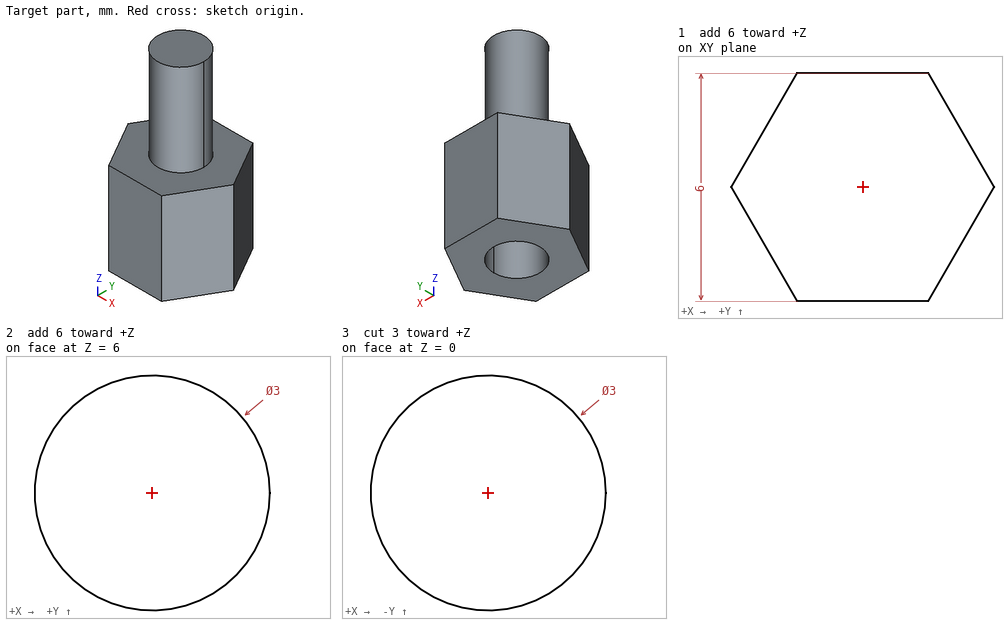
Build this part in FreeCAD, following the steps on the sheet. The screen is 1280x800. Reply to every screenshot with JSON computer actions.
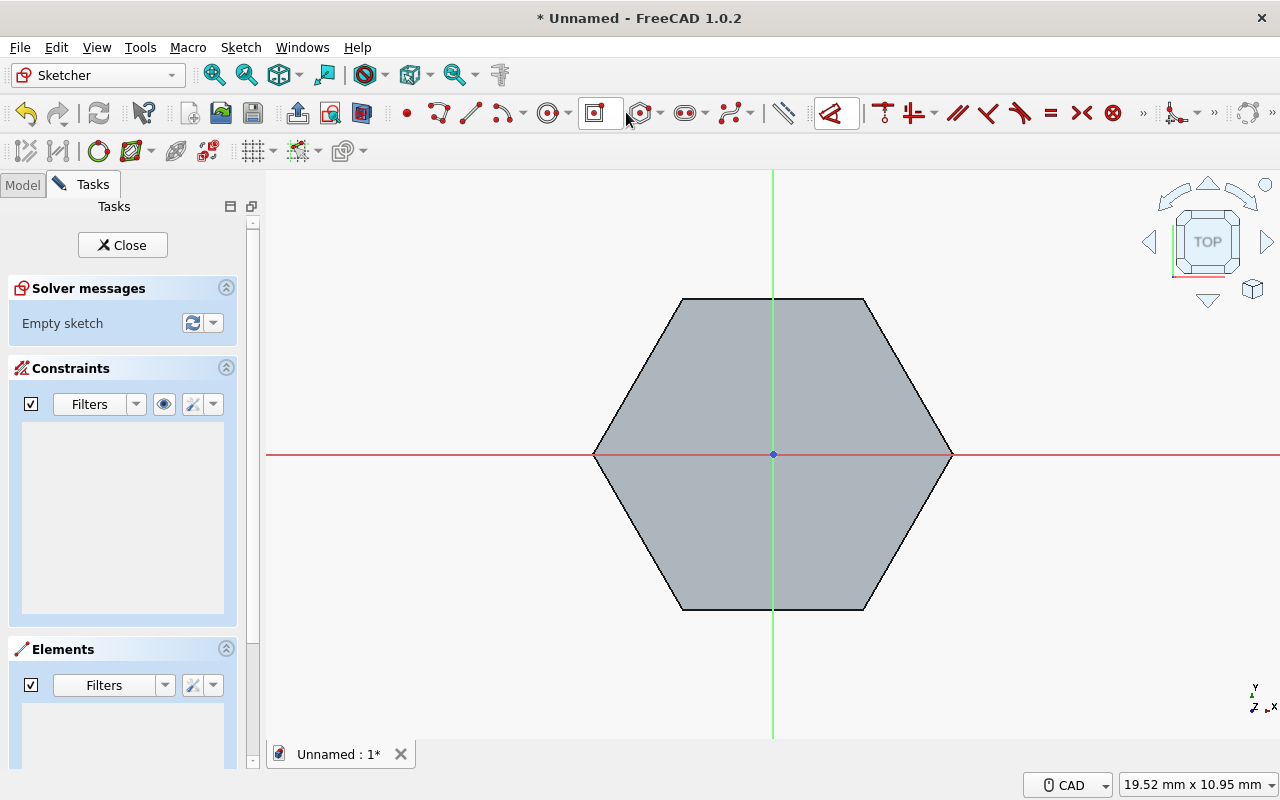
{"action": "scroll", "coordinate": [829, 455], "scroll_direction": "up", "scroll_amount": 4}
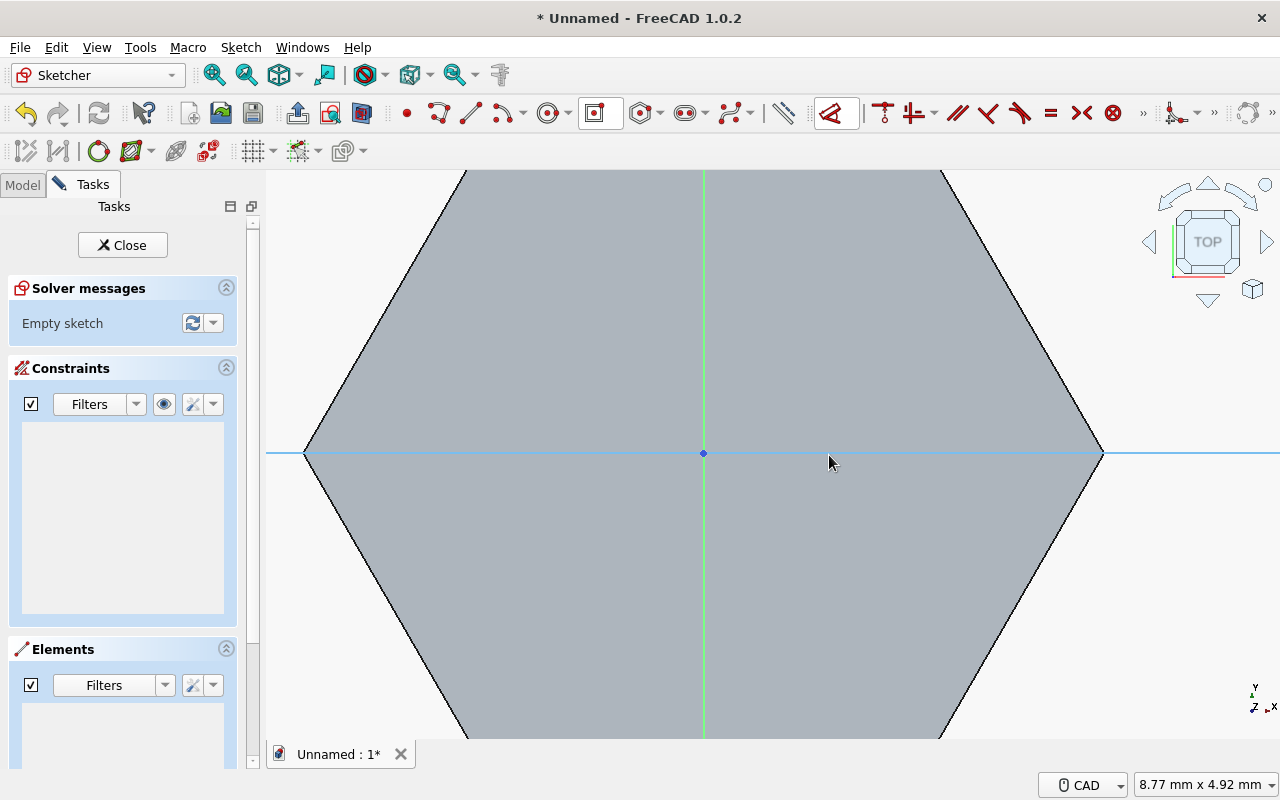
{"action": "left_click", "coordinate": [548, 114]}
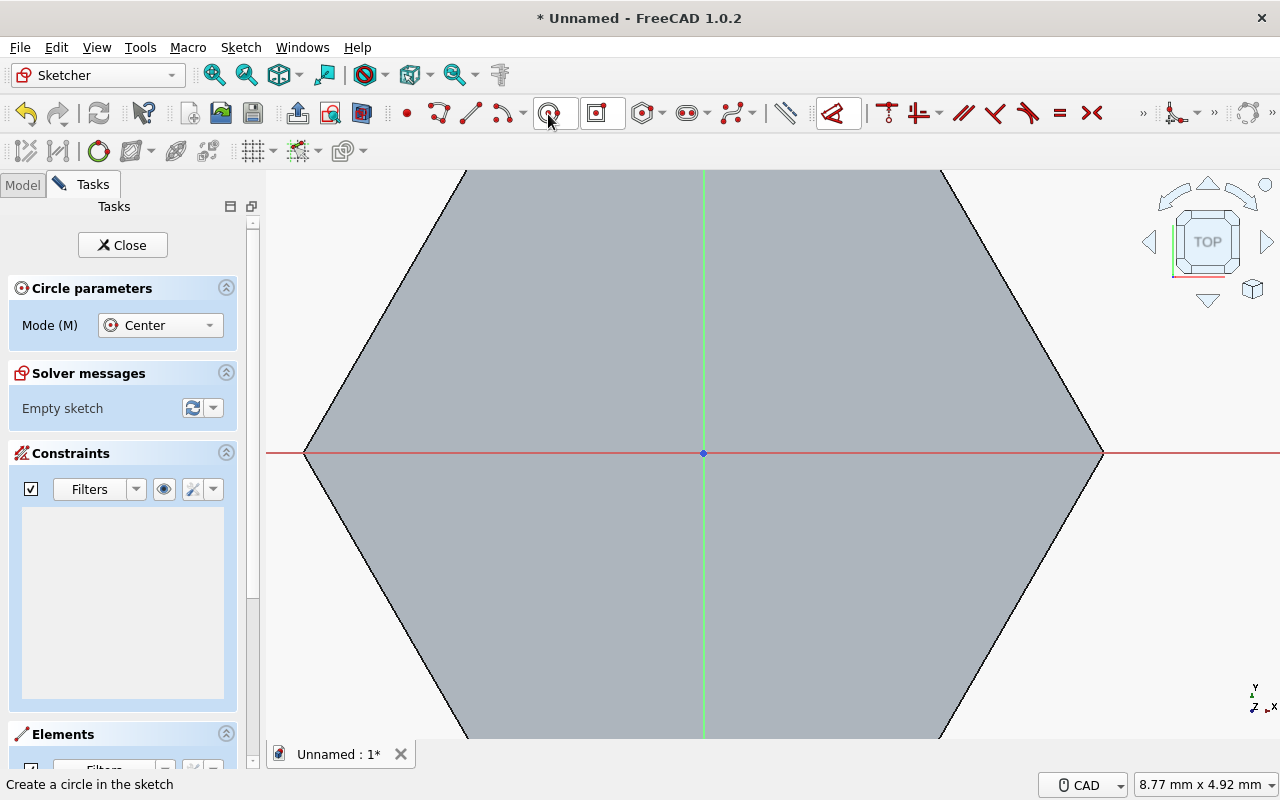
{"action": "left_click", "coordinate": [704, 453]}
{"action": "left_click", "coordinate": [826, 331]}
{"action": "key", "text": "Escape"}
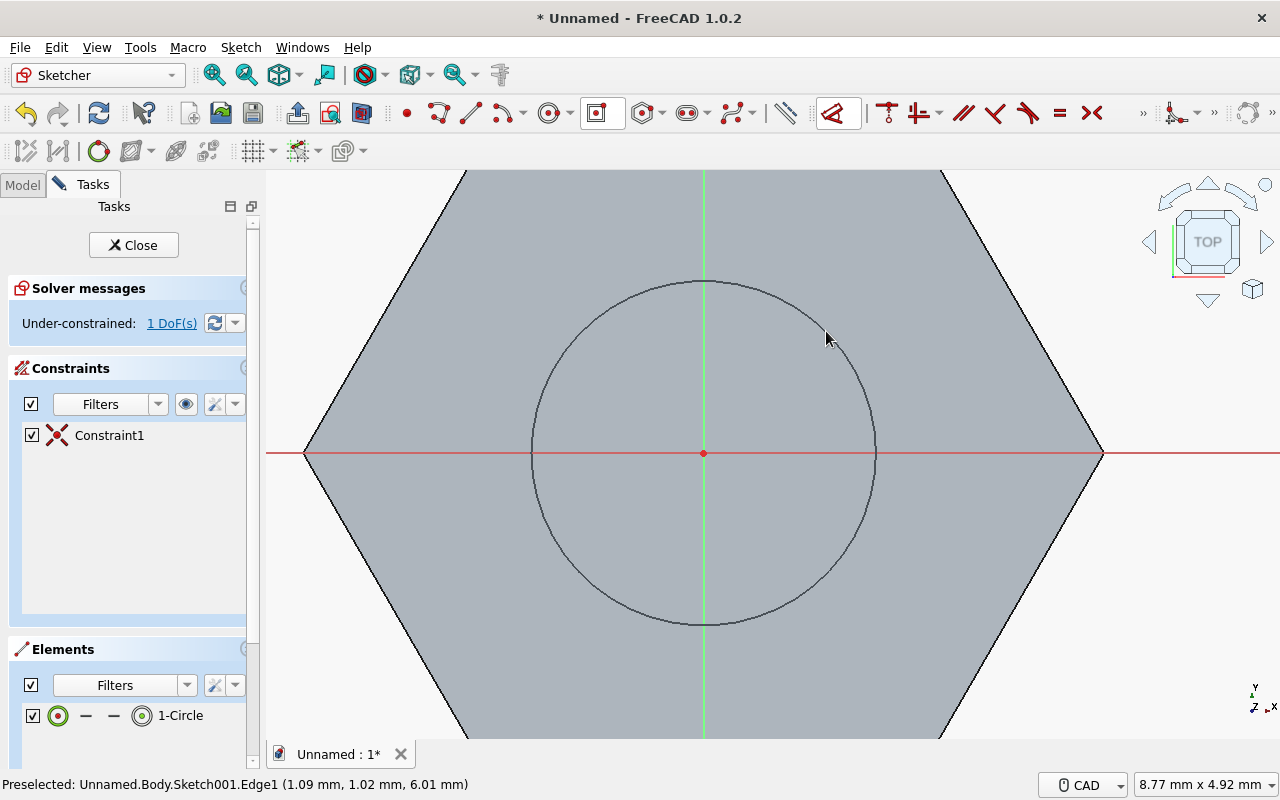
{"action": "left_click", "coordinate": [825, 331]}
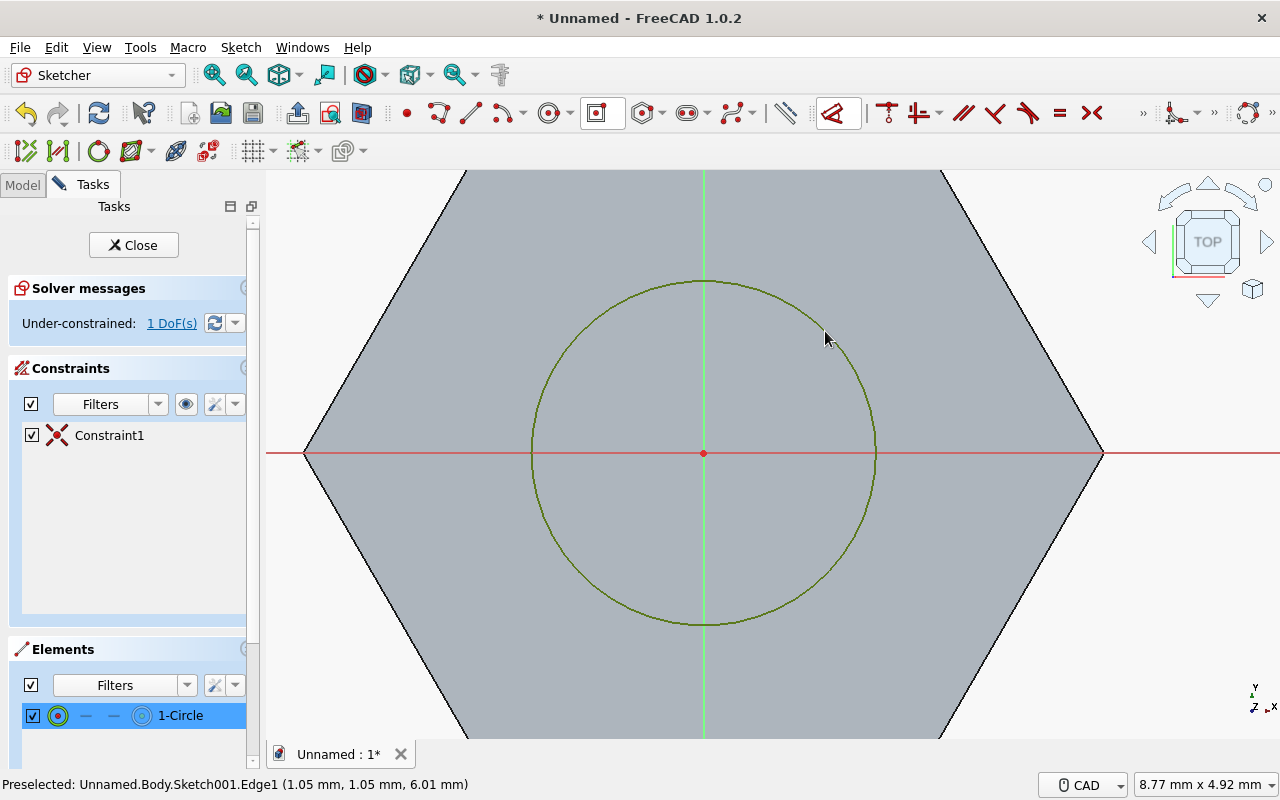
{"action": "left_click", "coordinate": [856, 114]}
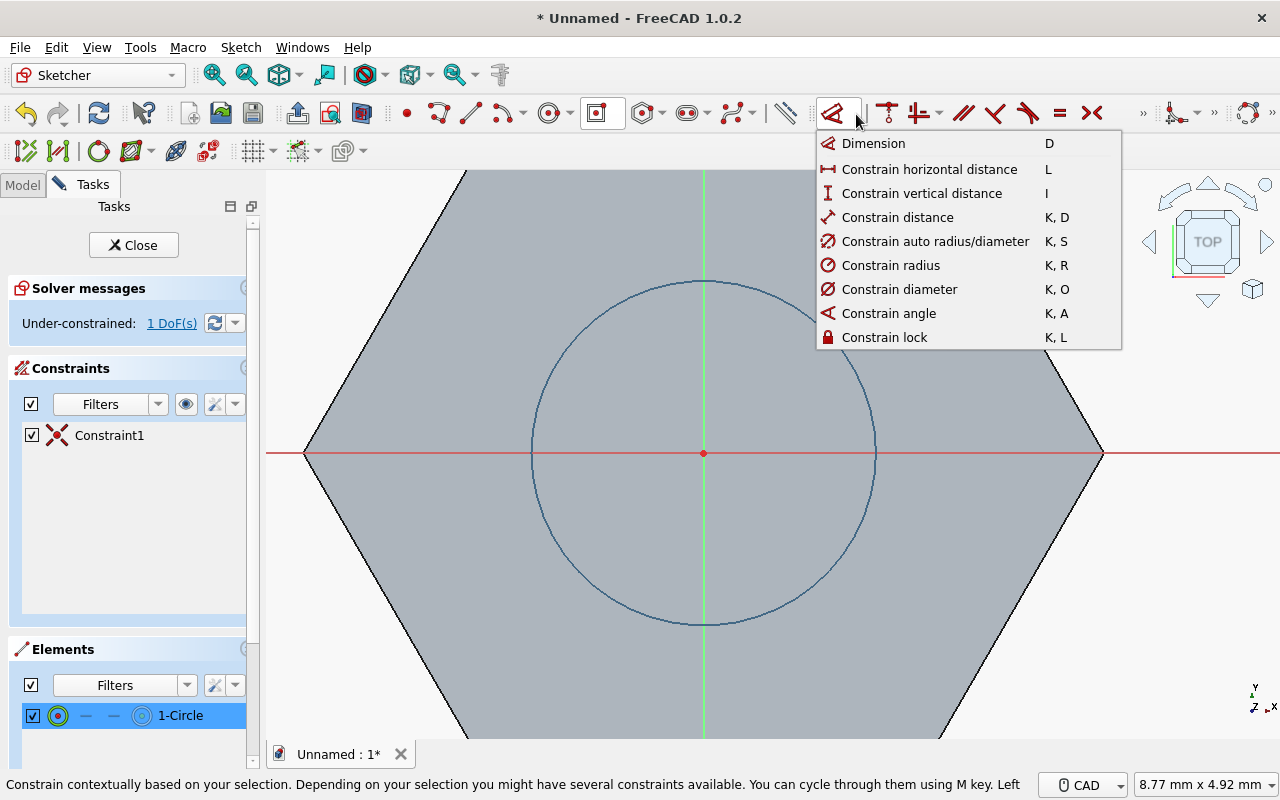
{"action": "left_click", "coordinate": [969, 289]}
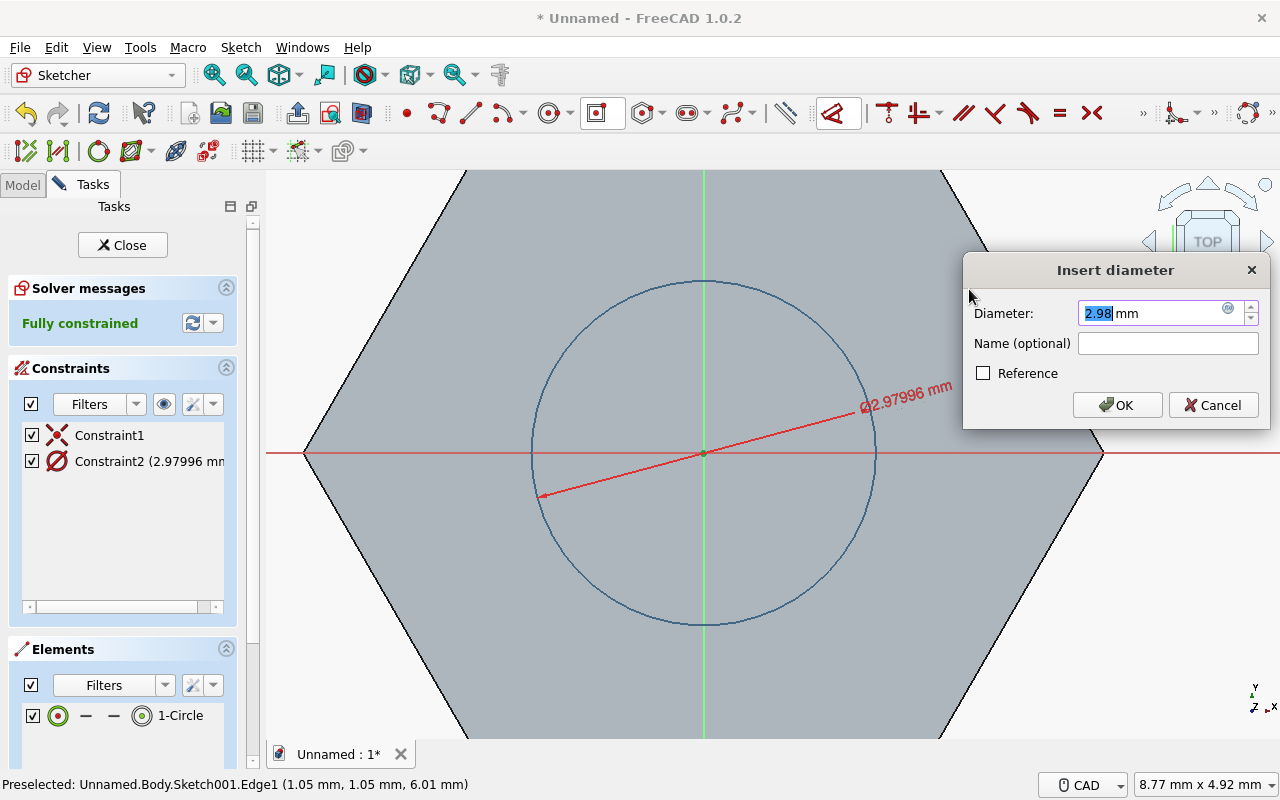
{"action": "type", "text": "3"}
{"action": "key", "text": "Return"}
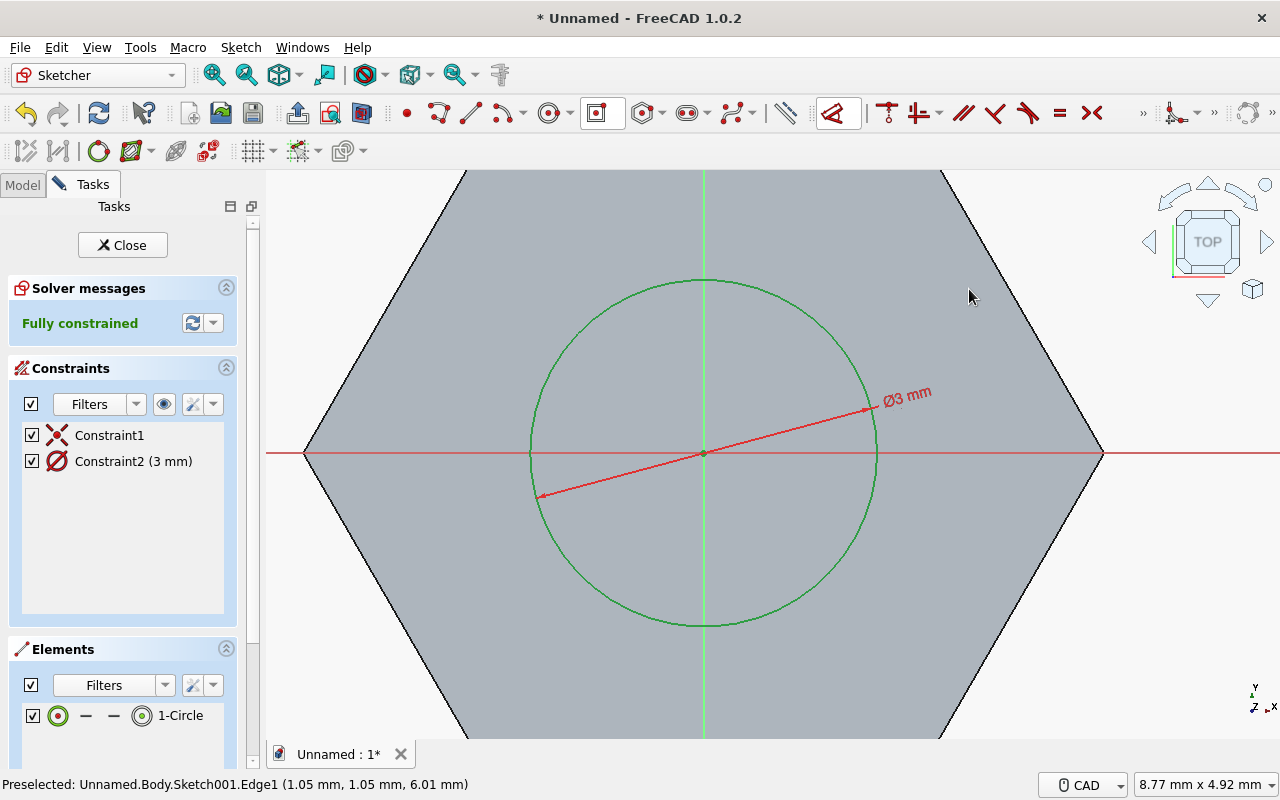
{"action": "left_click", "coordinate": [123, 245]}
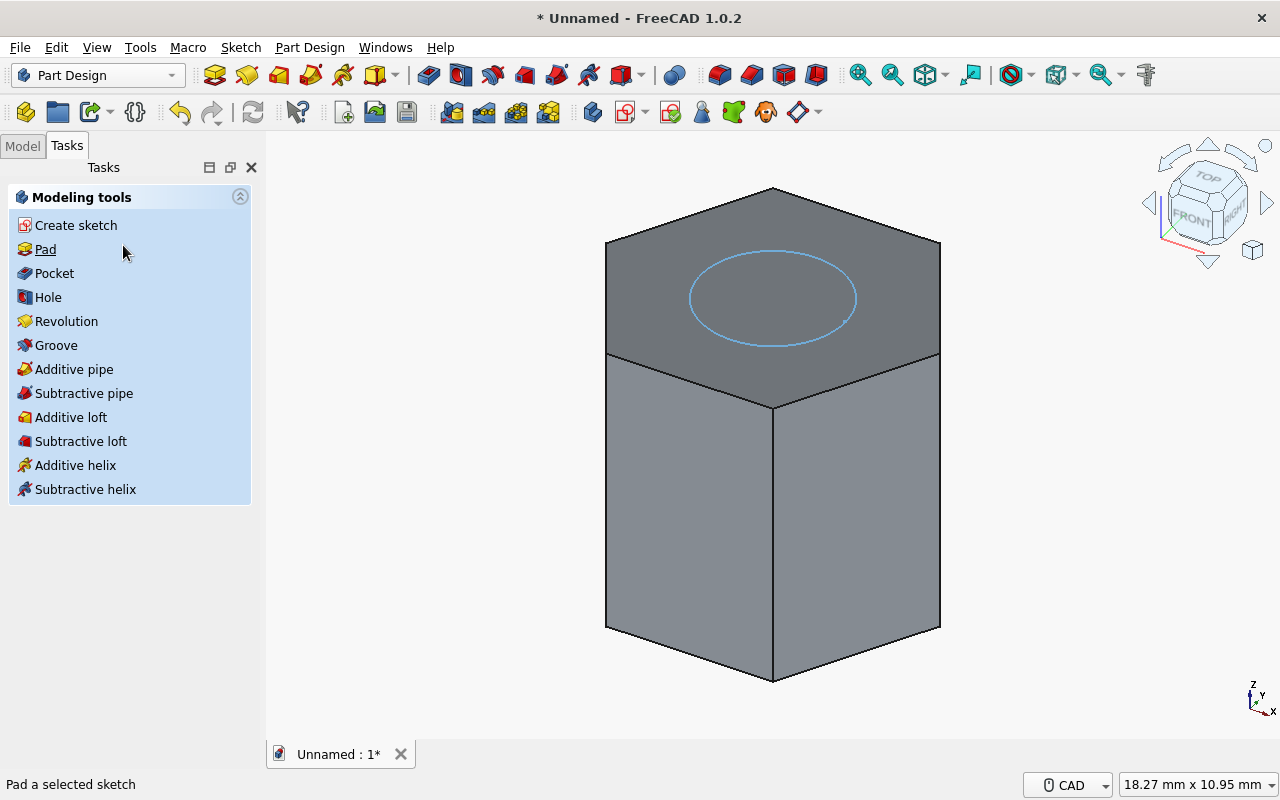
{"action": "left_click", "coordinate": [216, 76]}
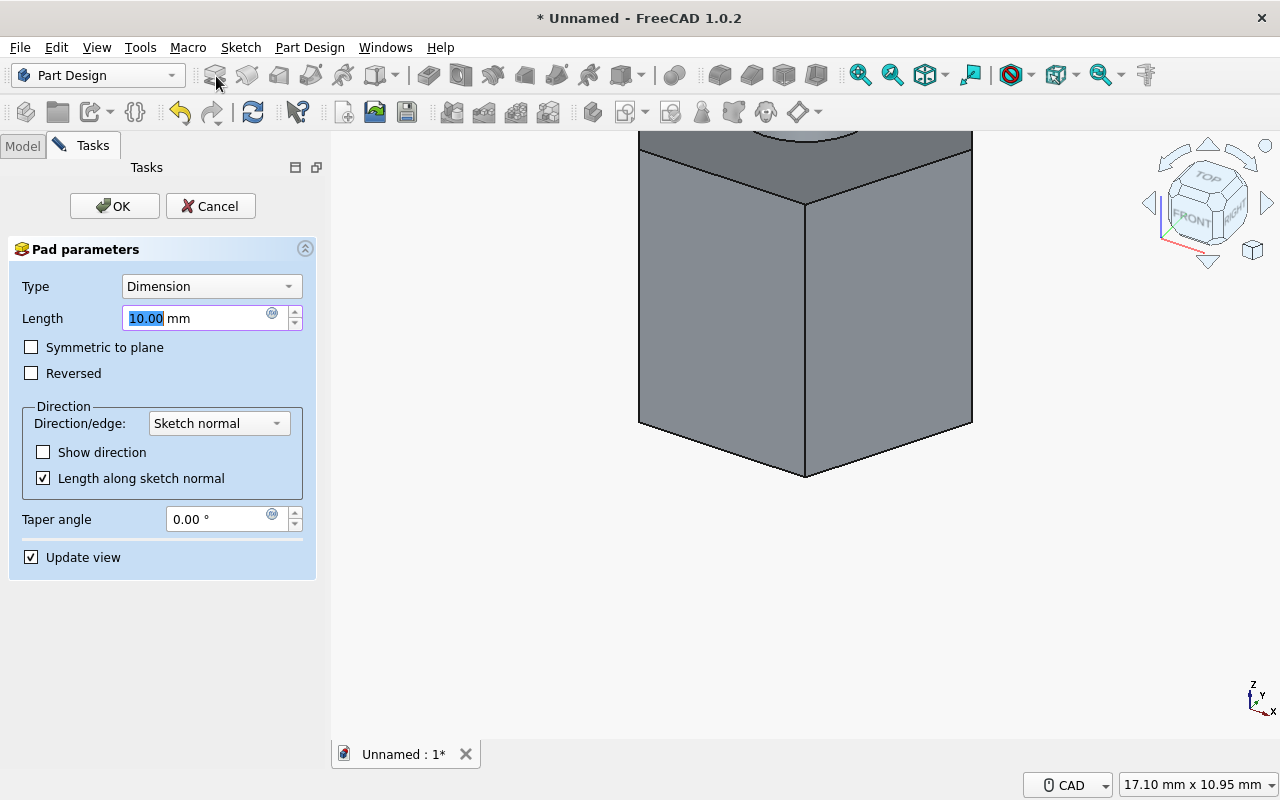
{"action": "type", "text": "6"}
{"action": "key", "text": "Tab"}